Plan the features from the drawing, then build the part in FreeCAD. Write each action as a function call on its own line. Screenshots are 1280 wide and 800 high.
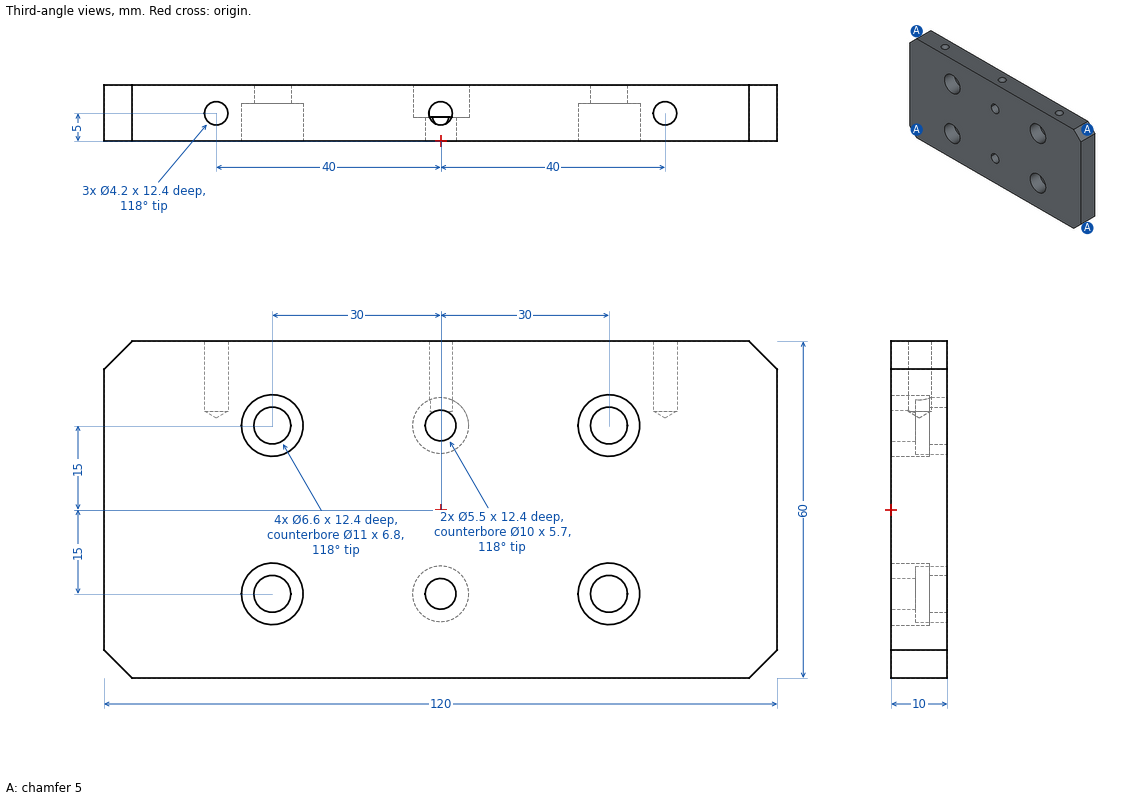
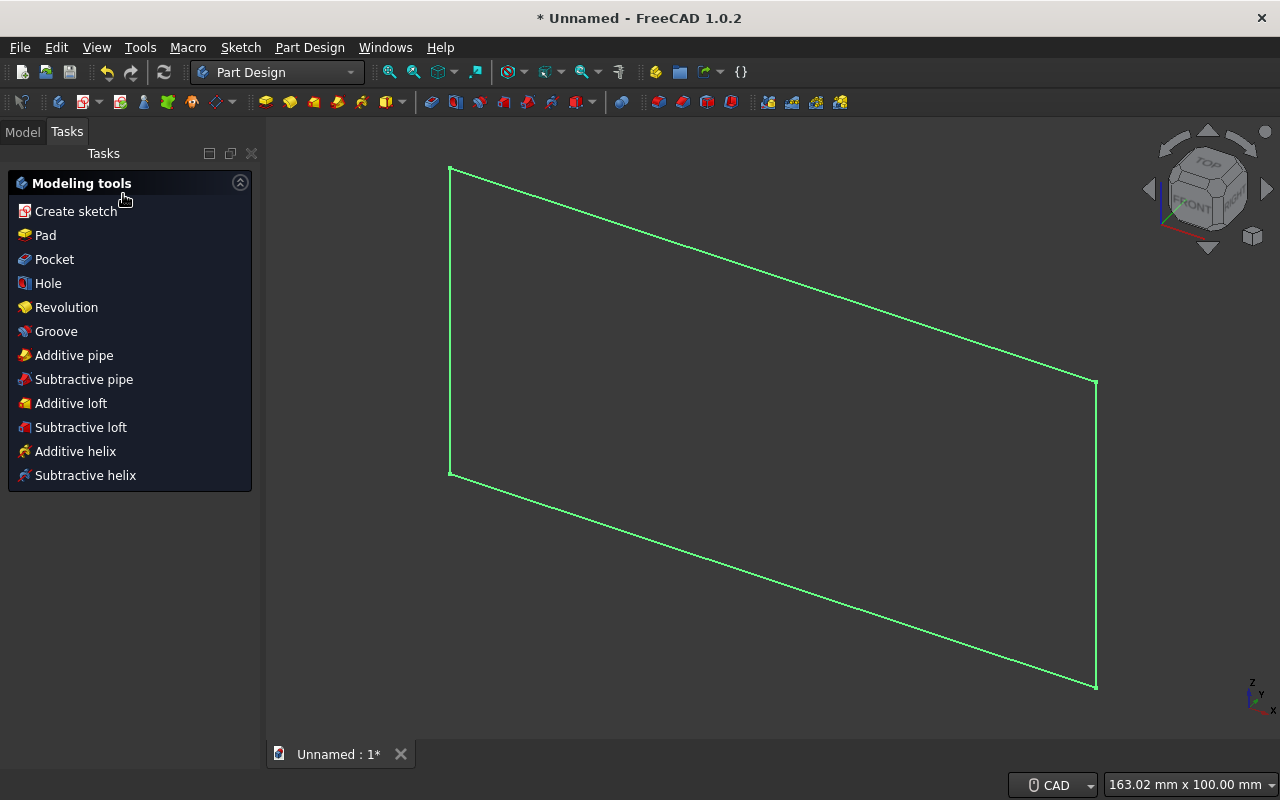
click(266, 102)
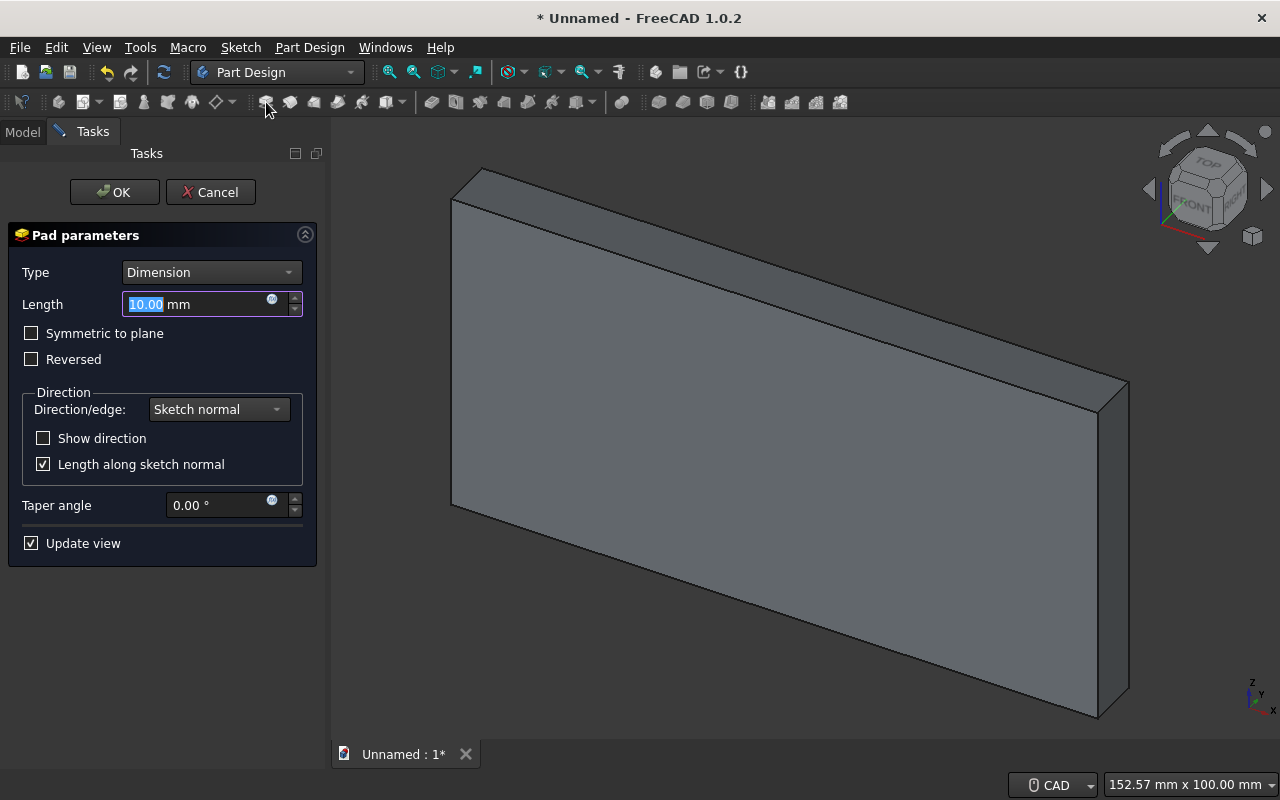
text(10)
key(Tab)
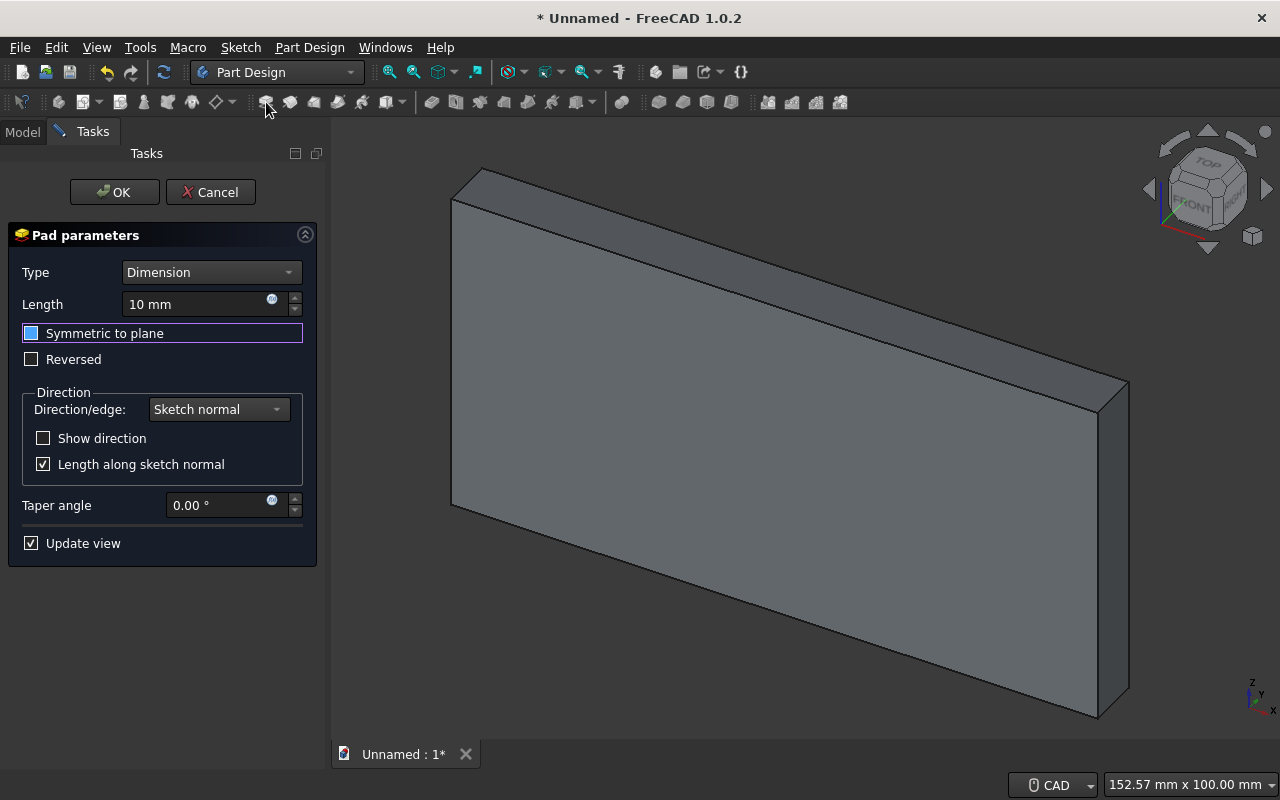
click(30, 359)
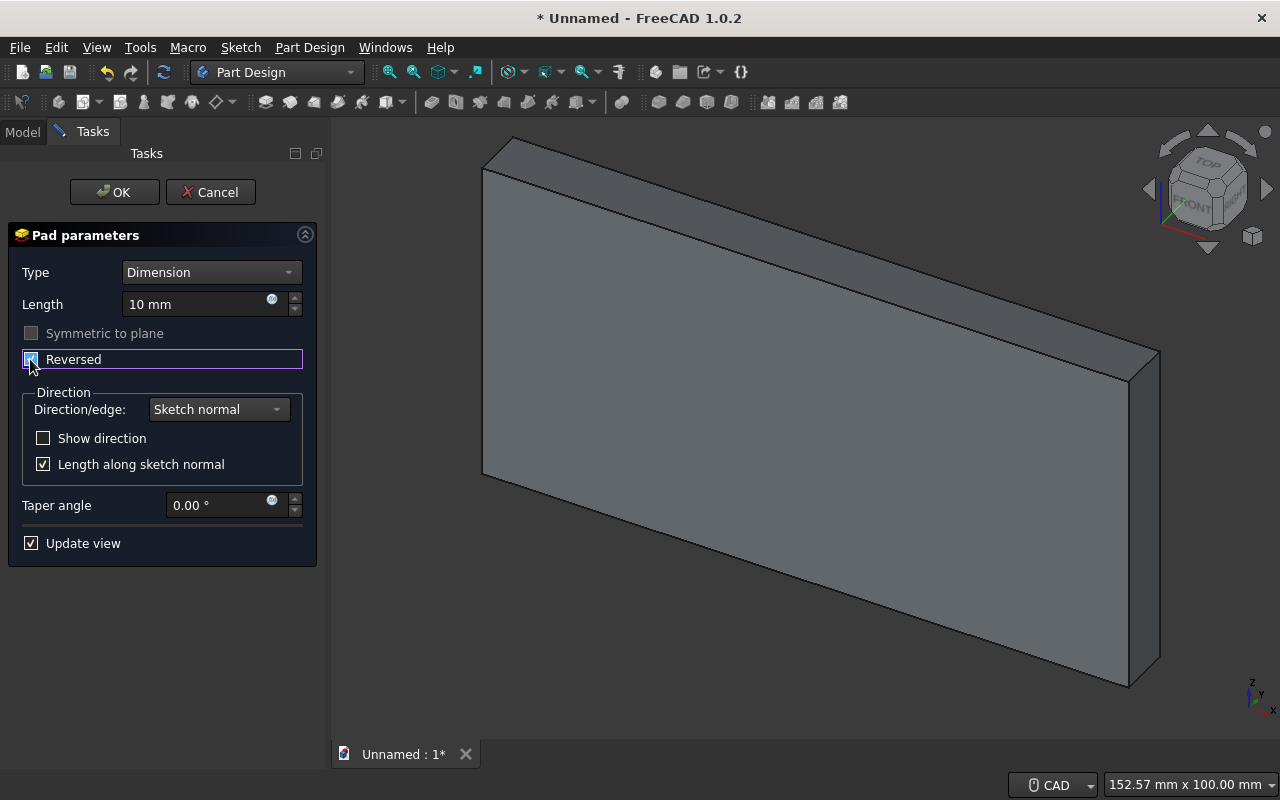
click(115, 192)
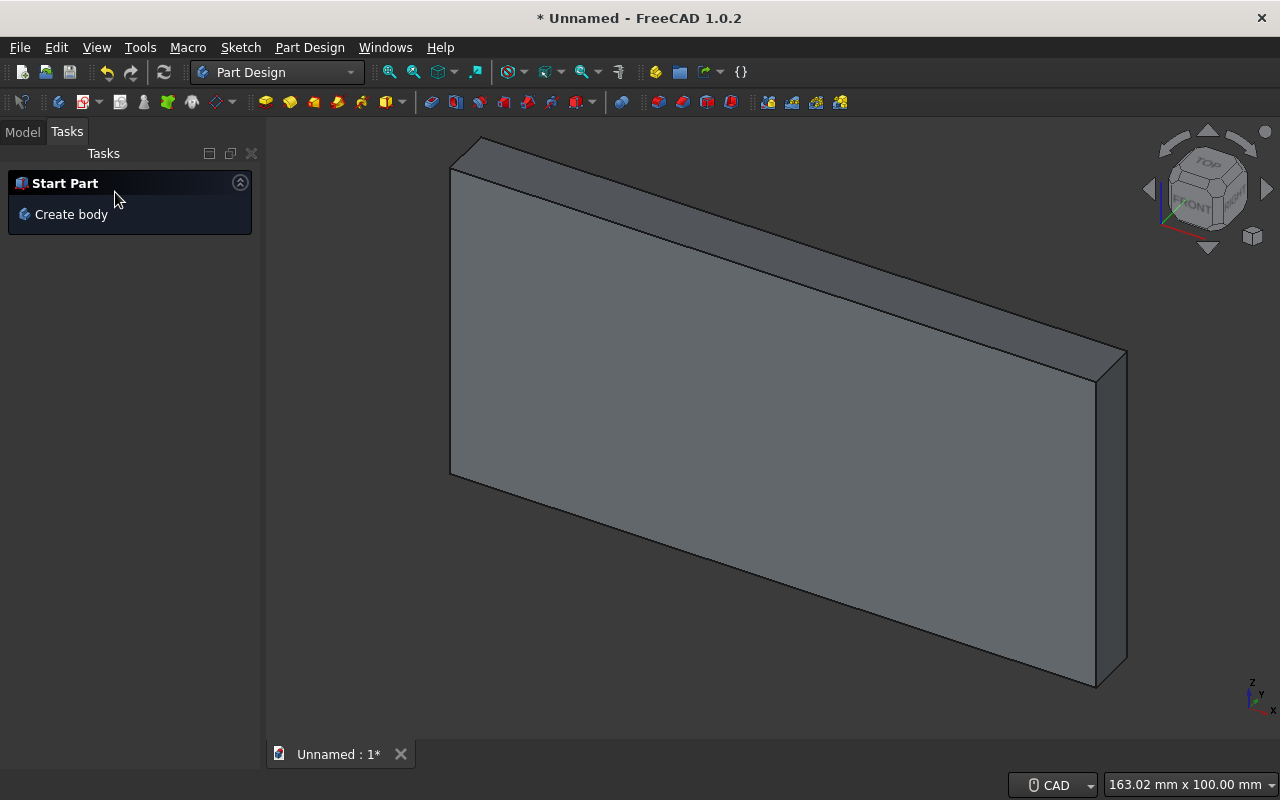
click(1112, 366)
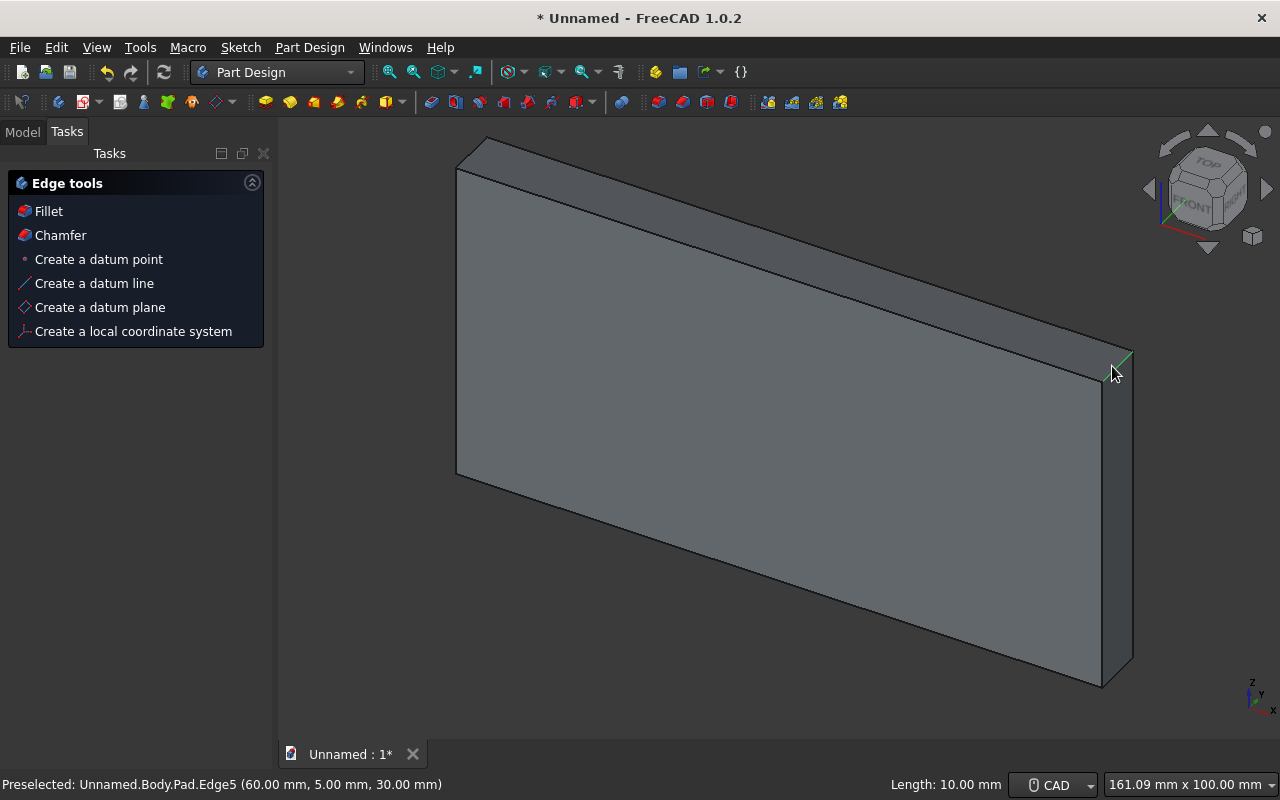
key(0)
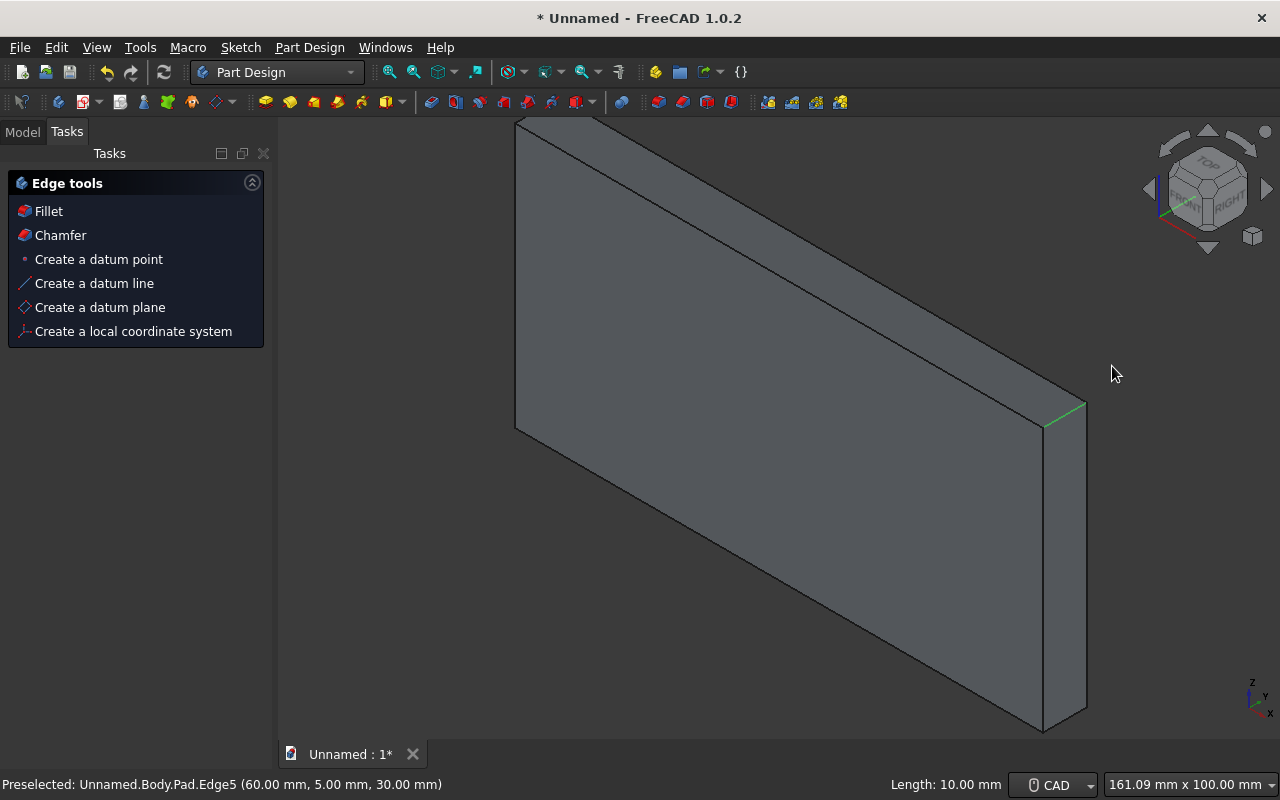
key(v)
key(f)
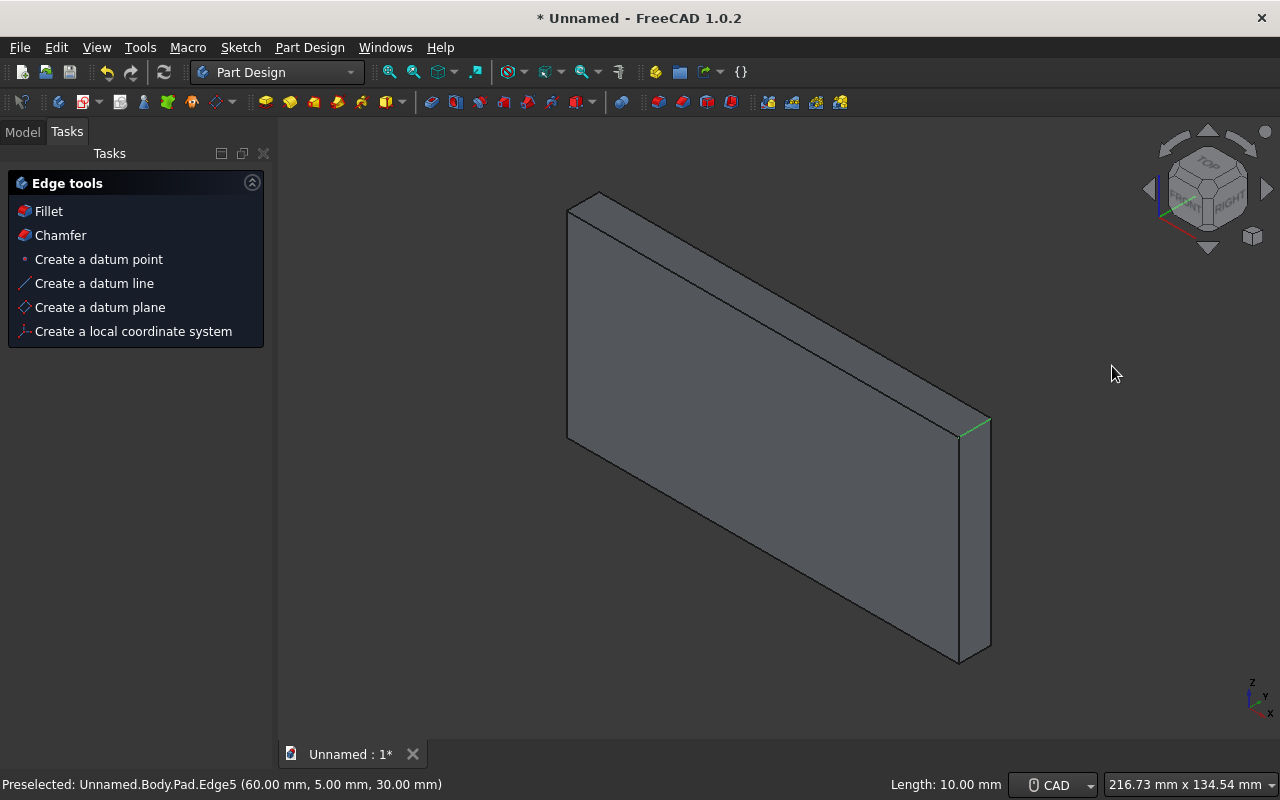
key(2)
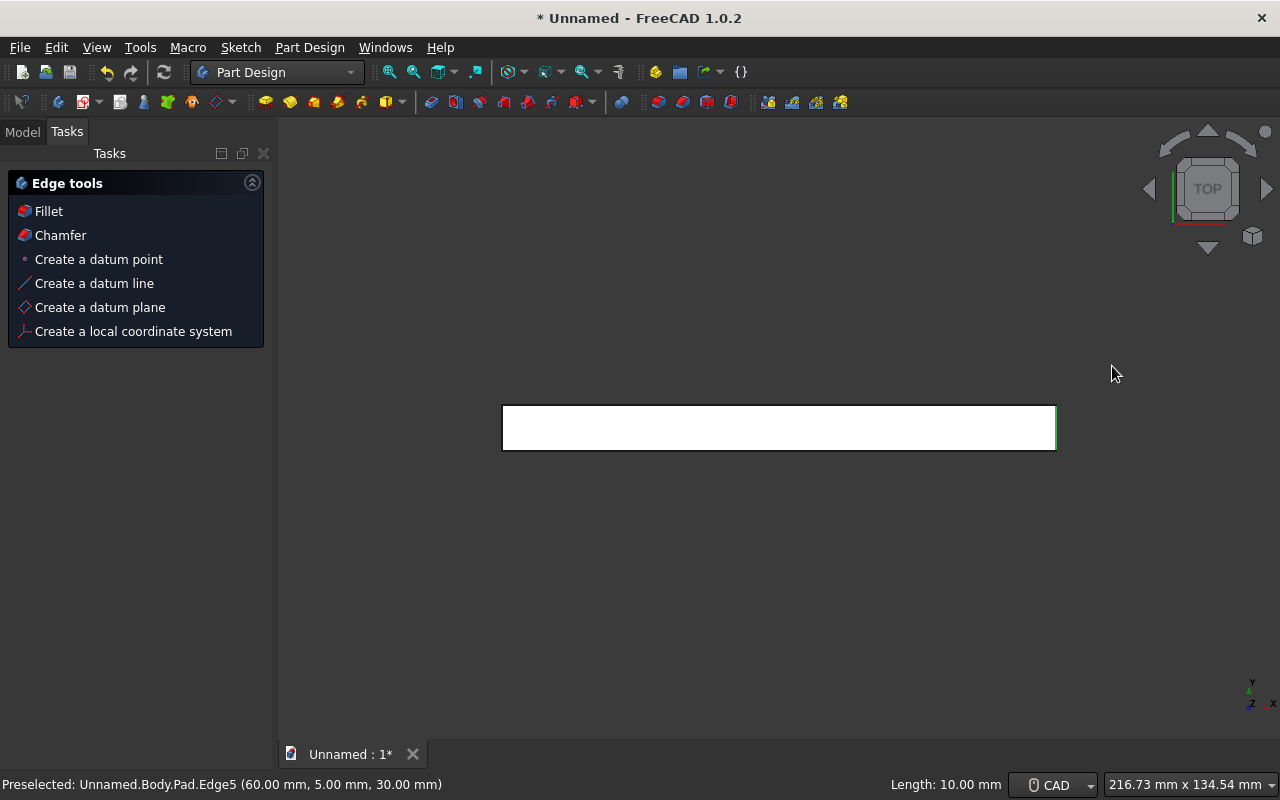
click(502, 427, ctrl)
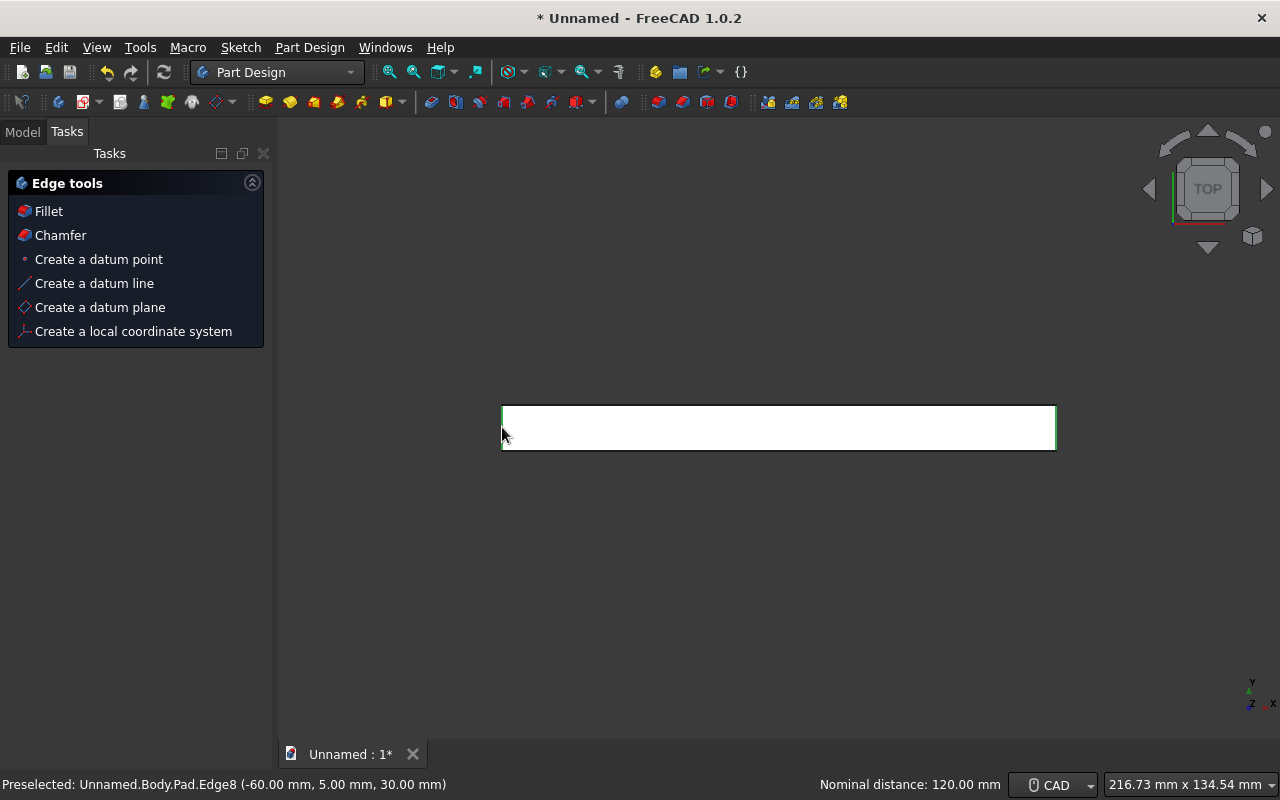
key(1)